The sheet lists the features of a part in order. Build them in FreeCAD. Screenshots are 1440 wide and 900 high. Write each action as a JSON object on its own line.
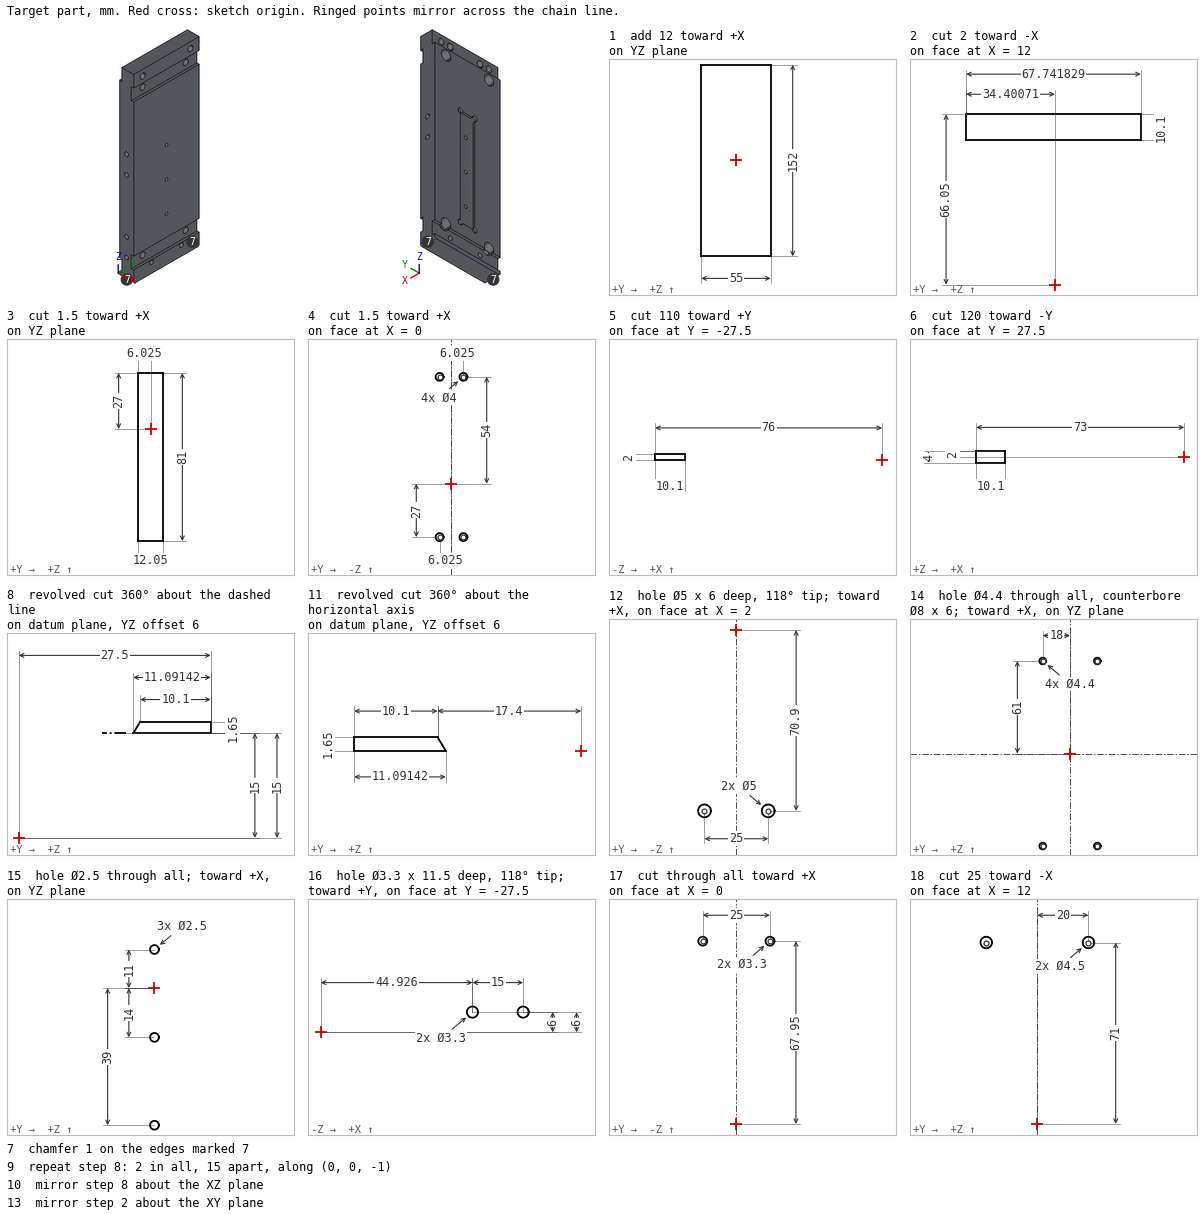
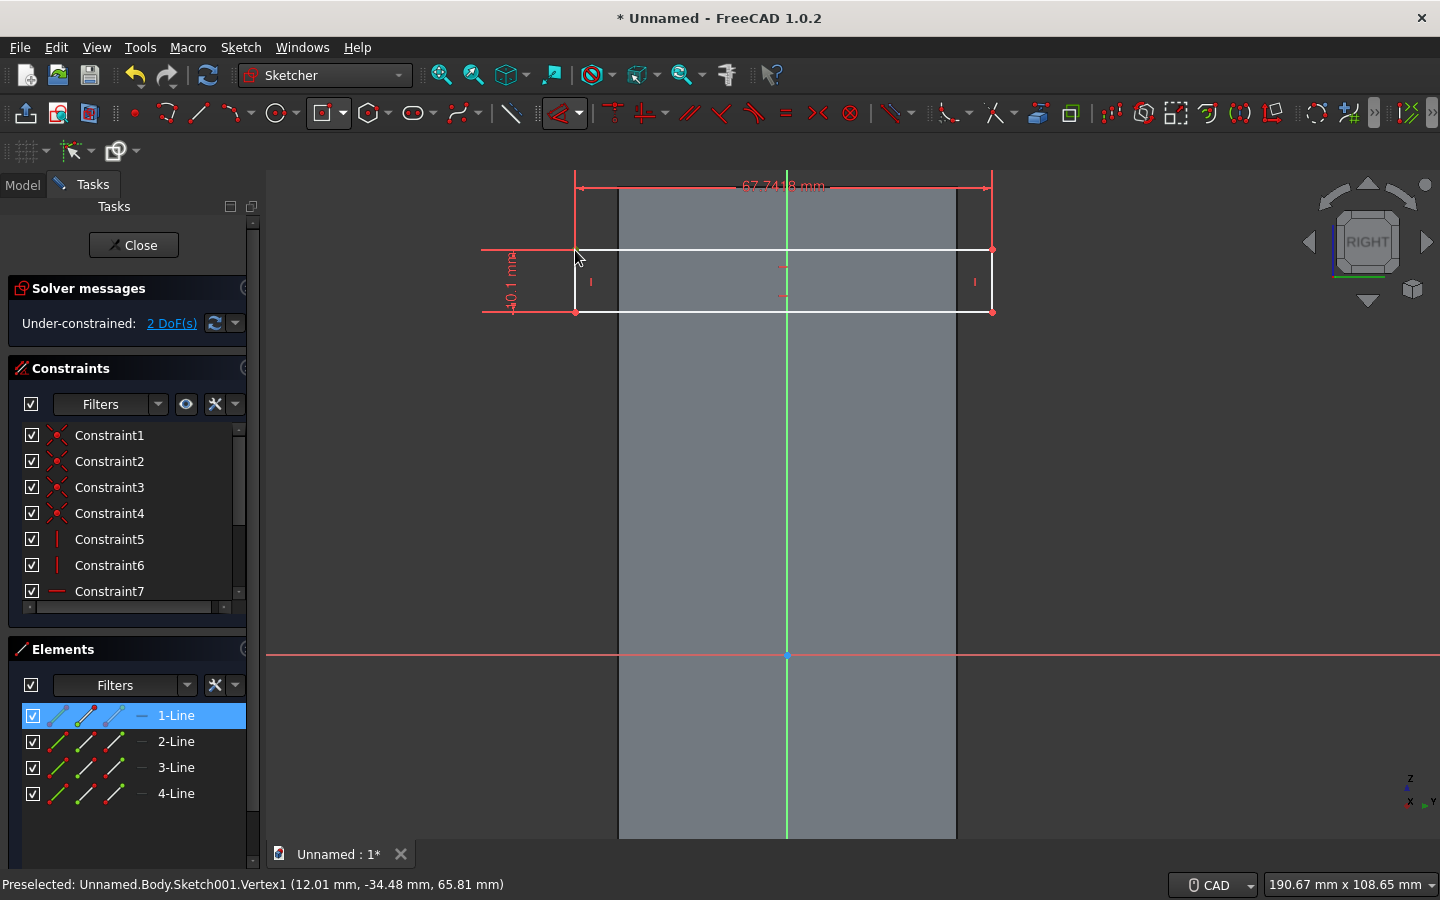
{"action": "key", "text": "i"}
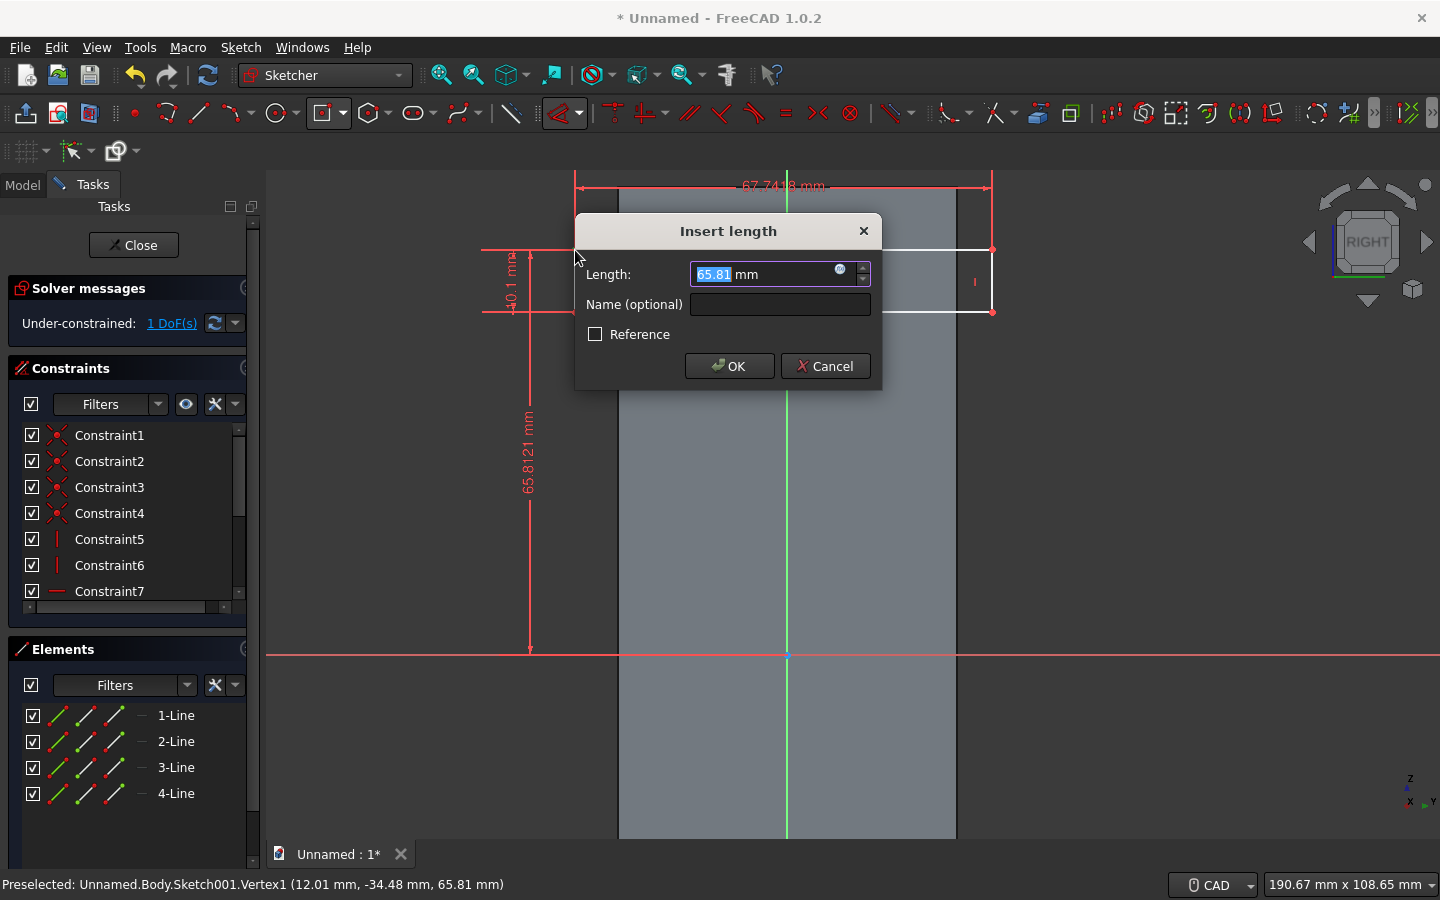
{"action": "type", "text": "66.05"}
{"action": "key", "text": "Return"}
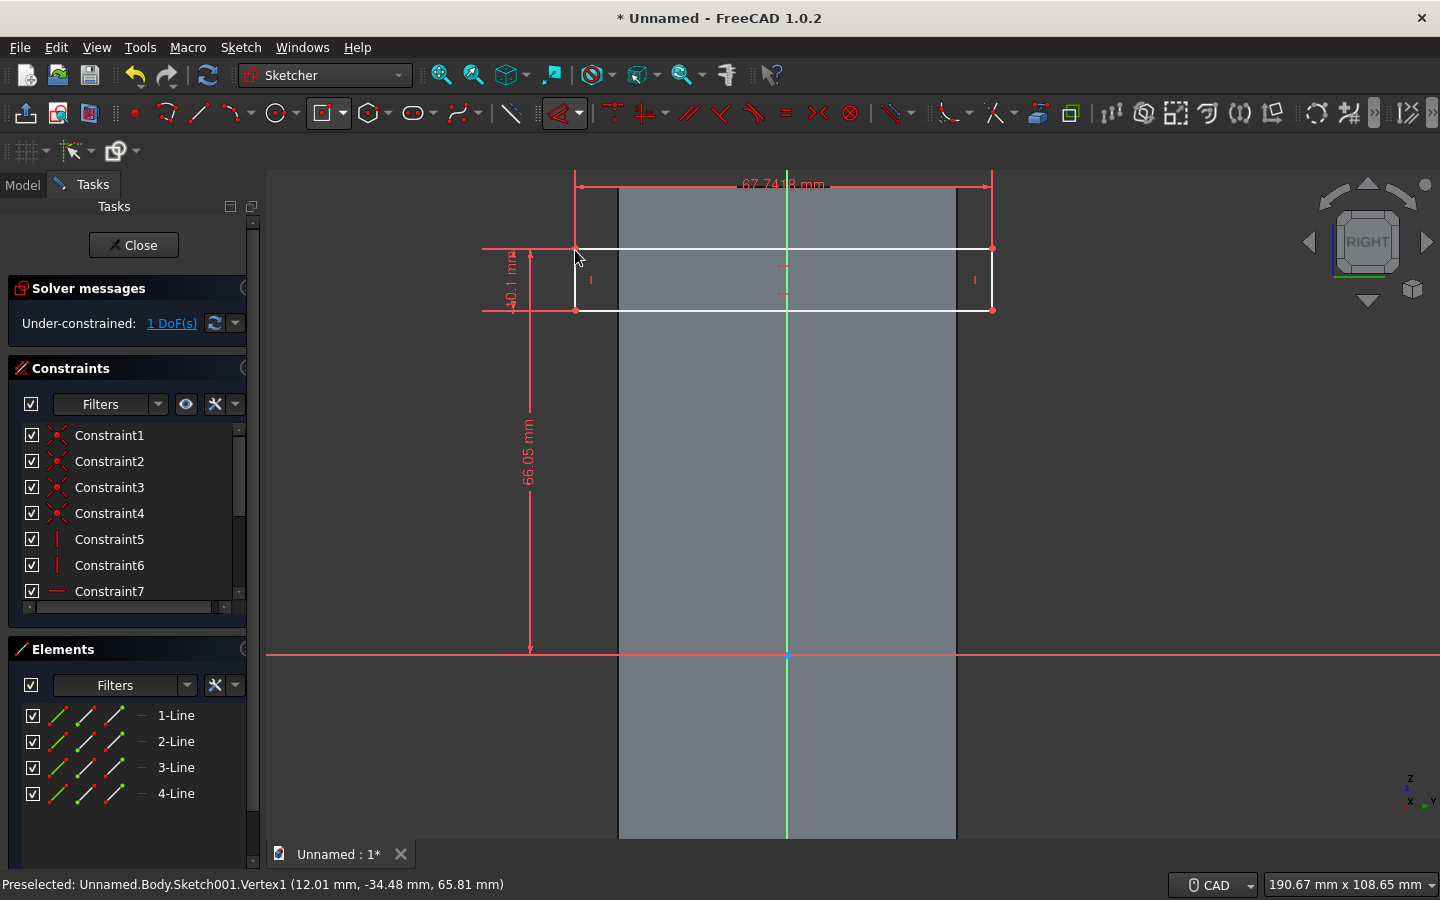
{"action": "left_click", "coordinate": [575, 249]}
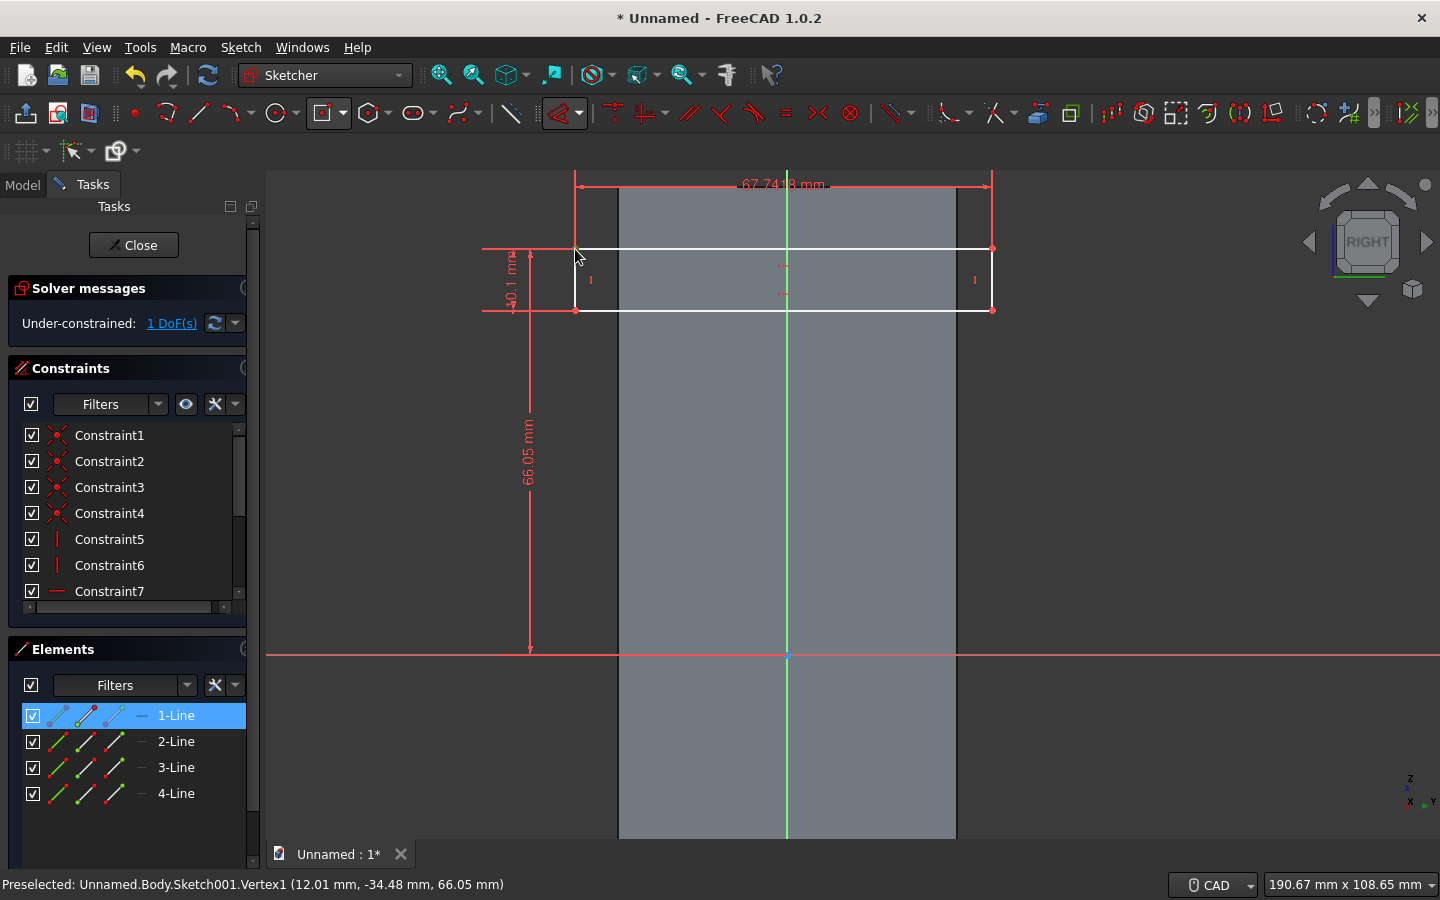
{"action": "left_click", "coordinate": [582, 114]}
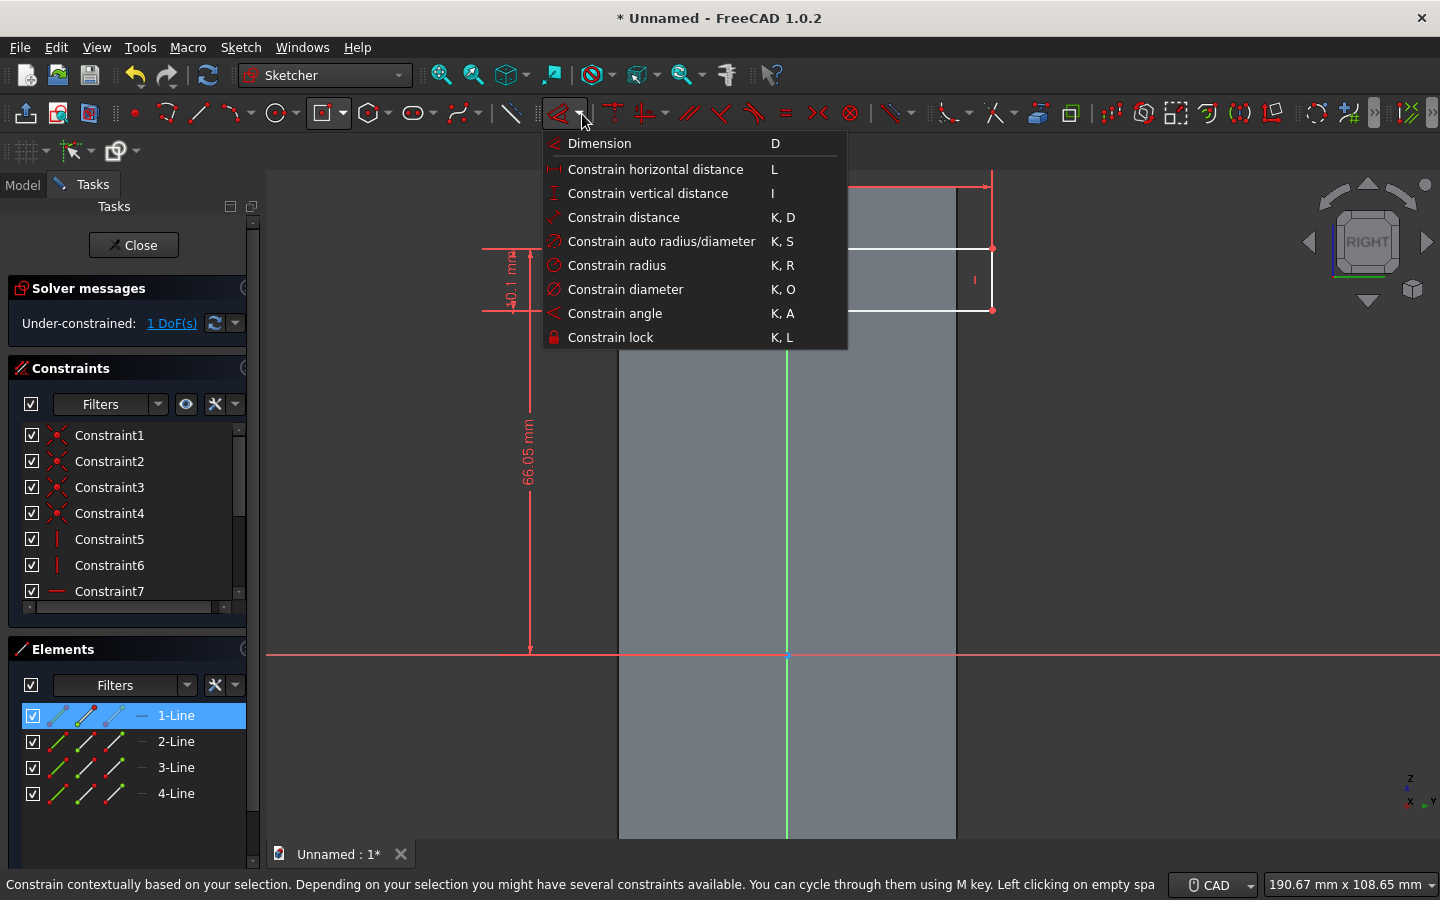
{"action": "left_click", "coordinate": [695, 169]}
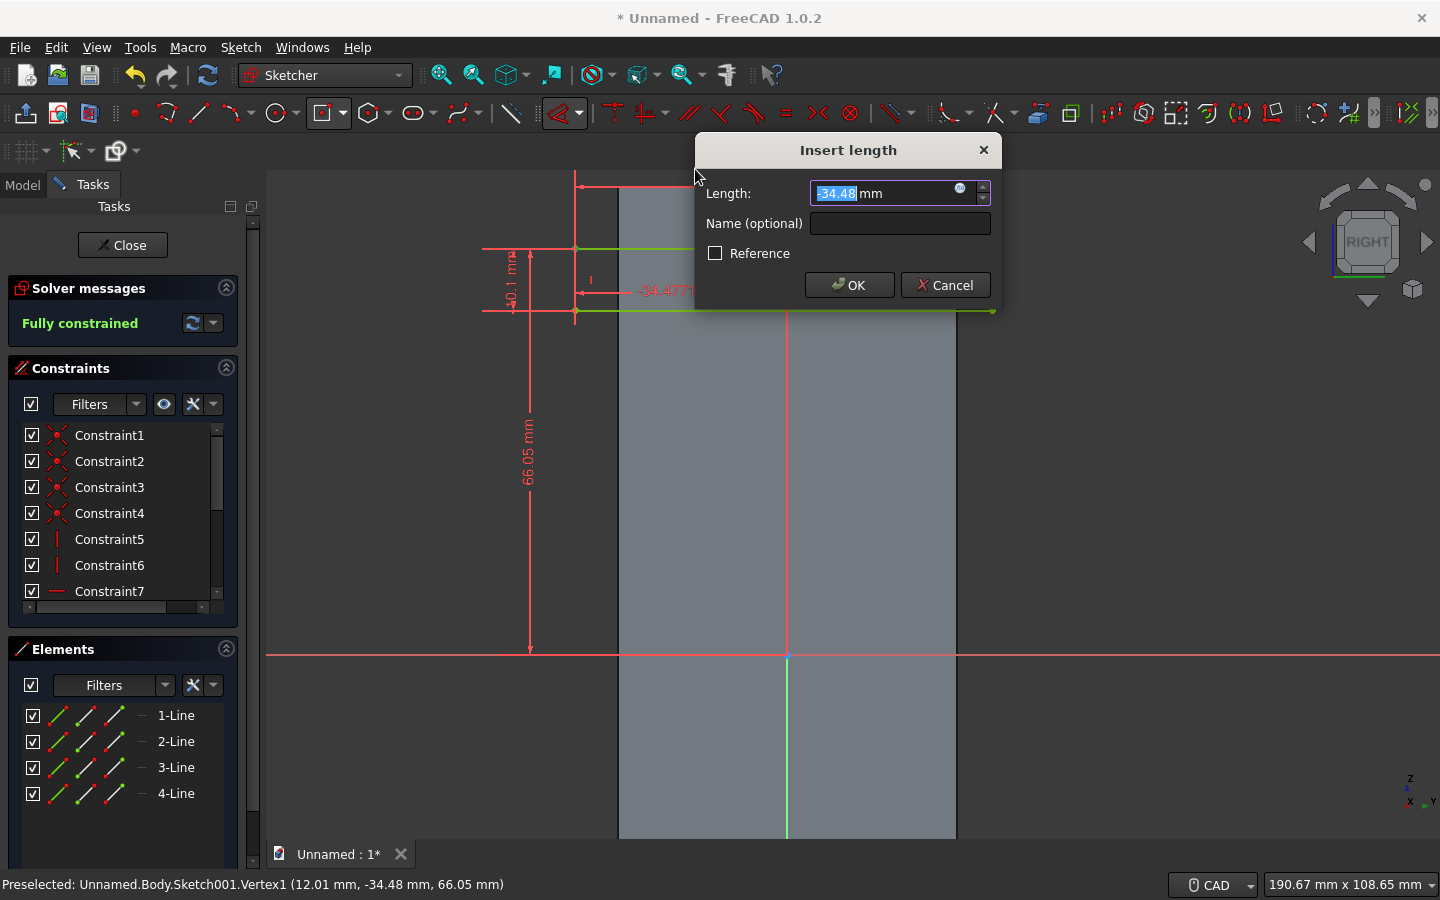
{"action": "type", "text": "-34.40071"}
{"action": "key", "text": "Return"}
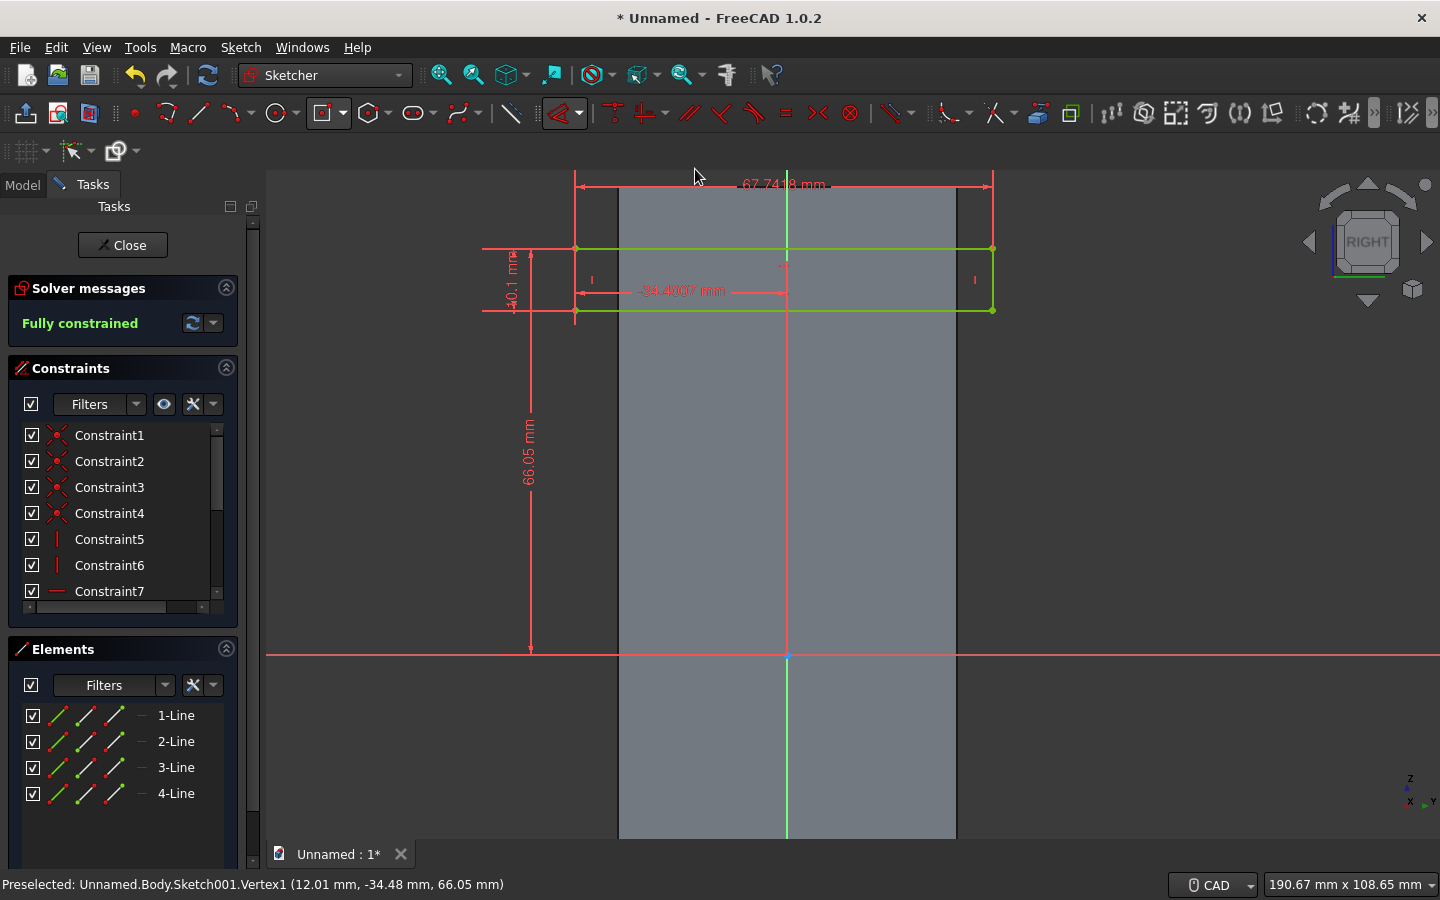
{"action": "left_click", "coordinate": [123, 245]}